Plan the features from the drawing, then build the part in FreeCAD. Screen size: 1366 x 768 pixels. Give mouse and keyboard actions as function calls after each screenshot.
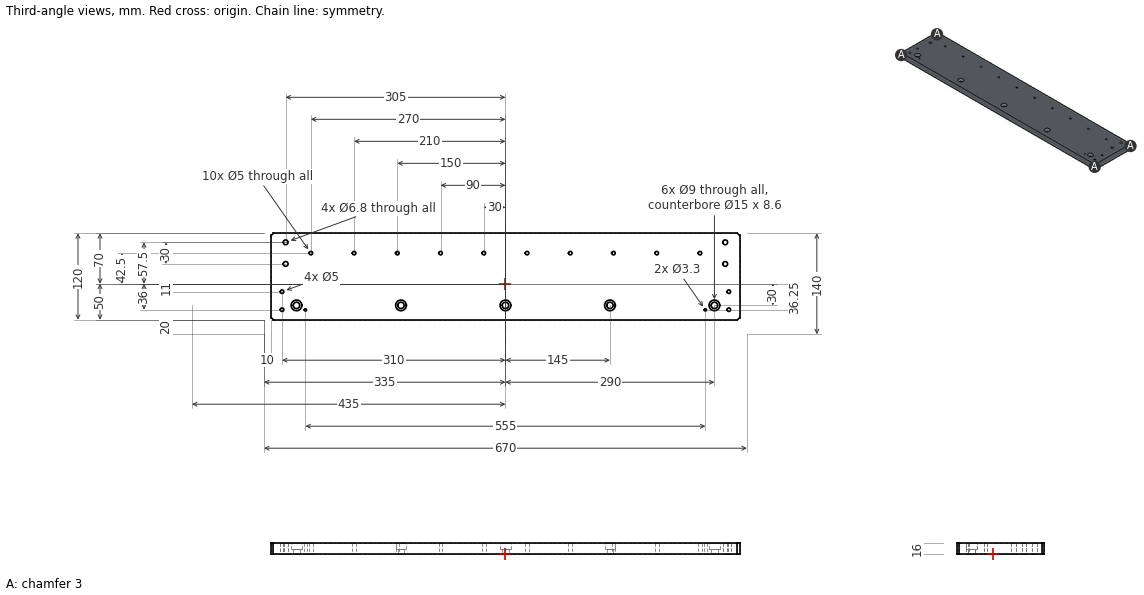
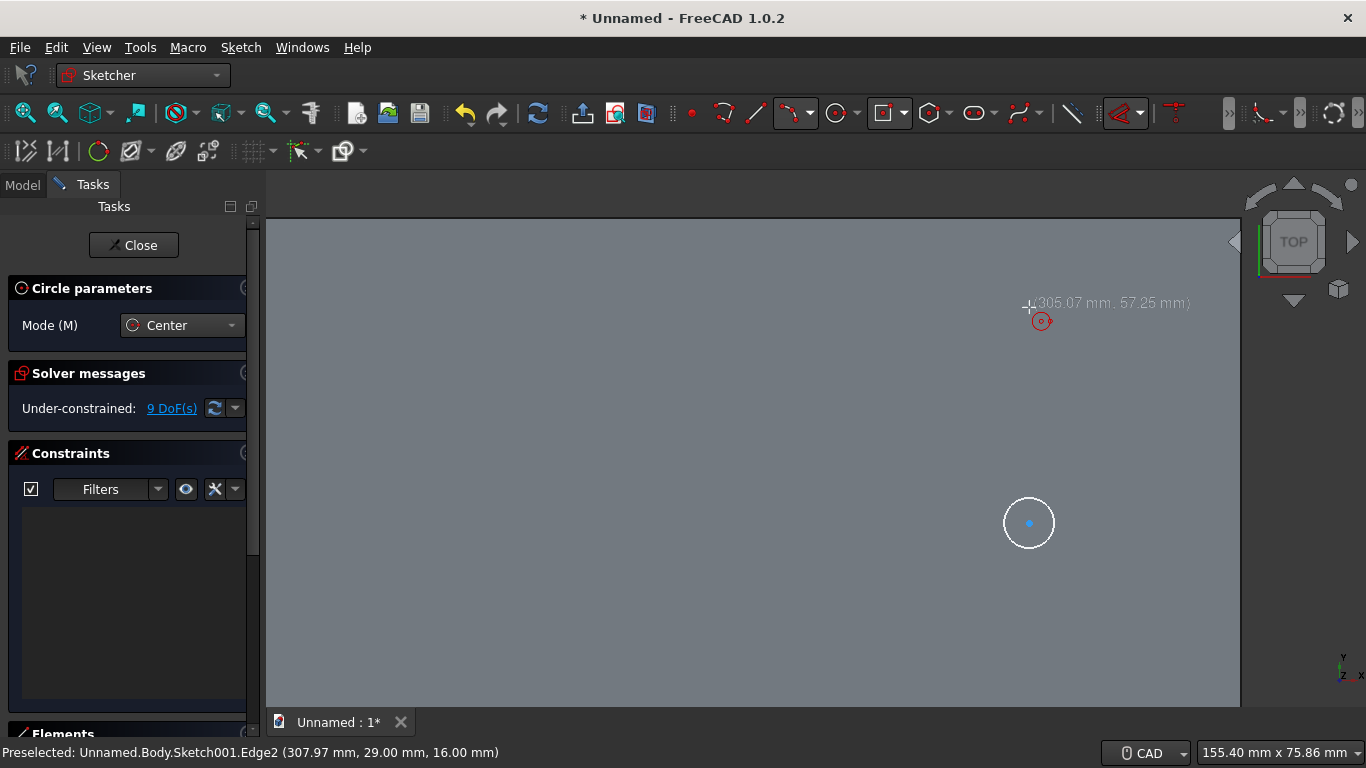
scroll(1041, 429, down, 10)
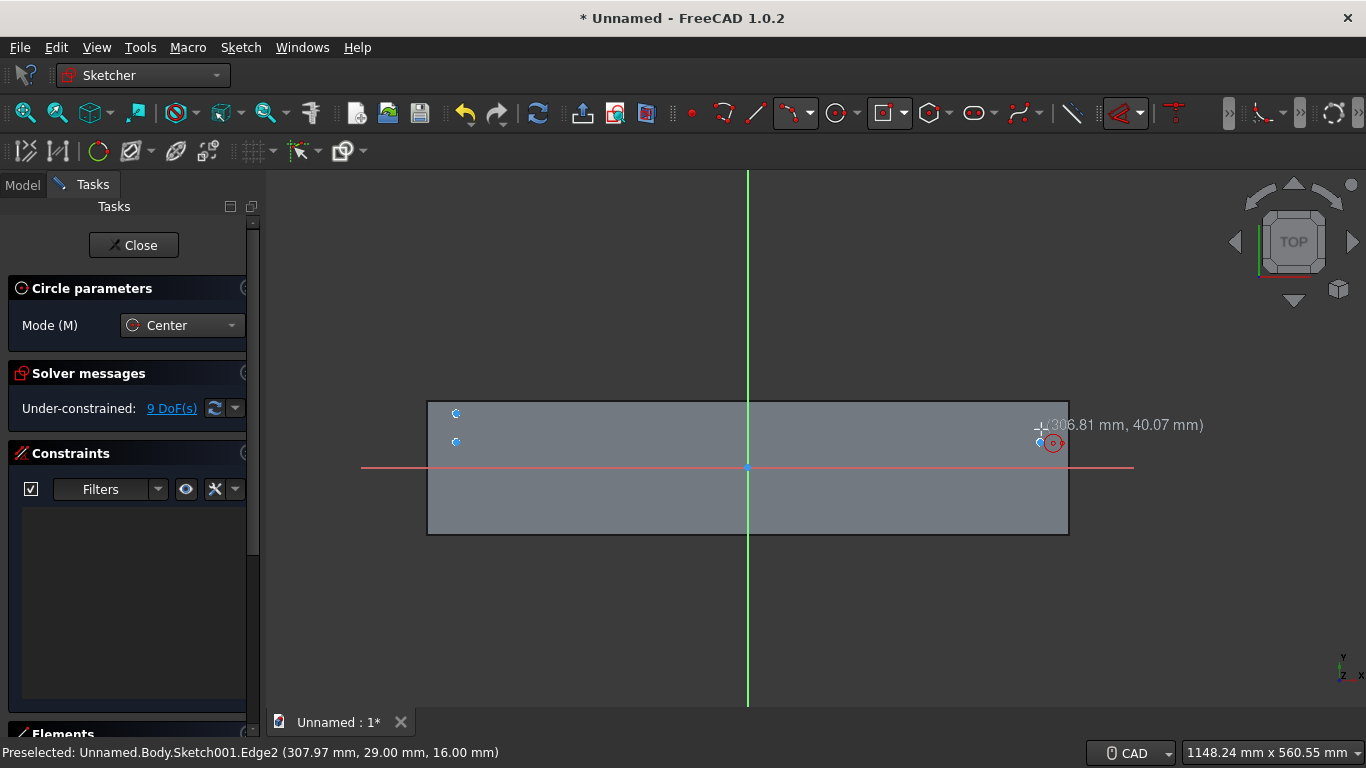
click(1040, 413)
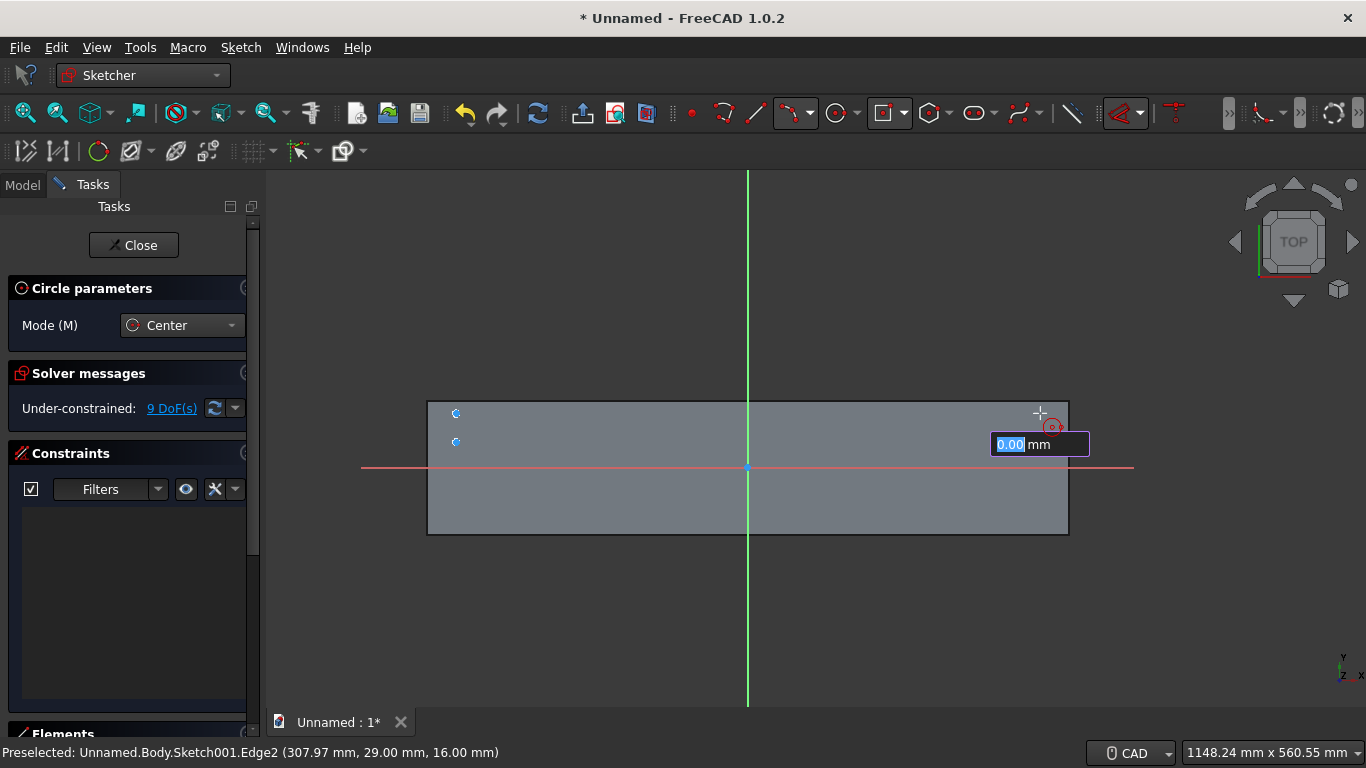
scroll(1042, 411, up, 8)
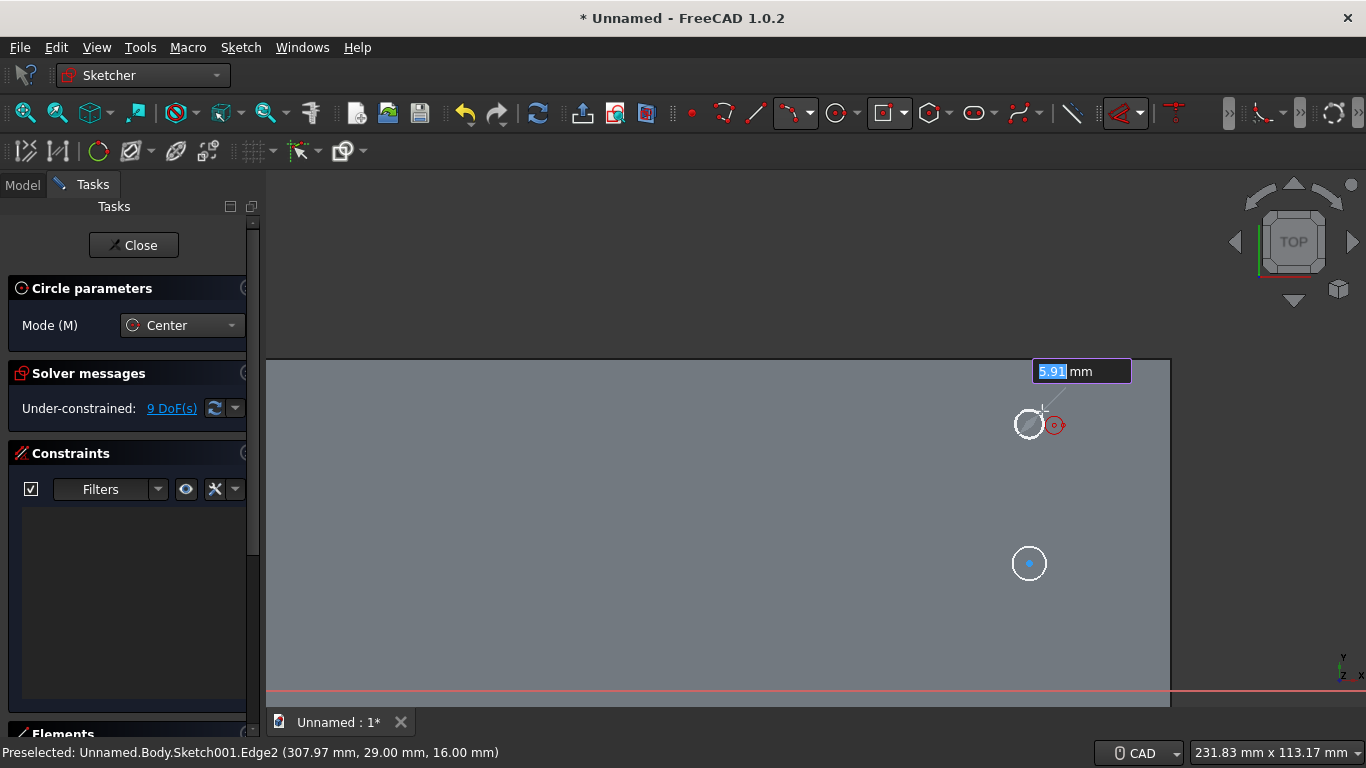
click(1040, 407)
key(Escape)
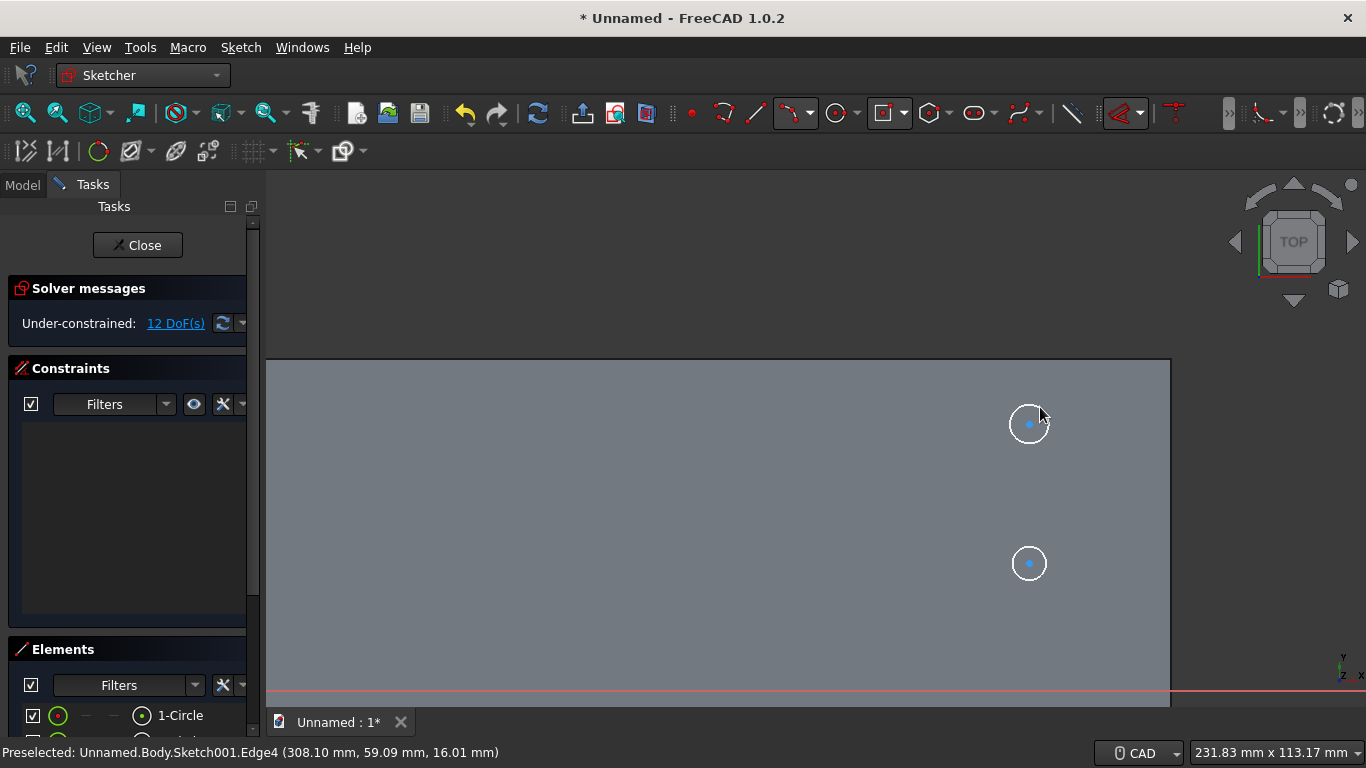
scroll(1042, 411, down, 8)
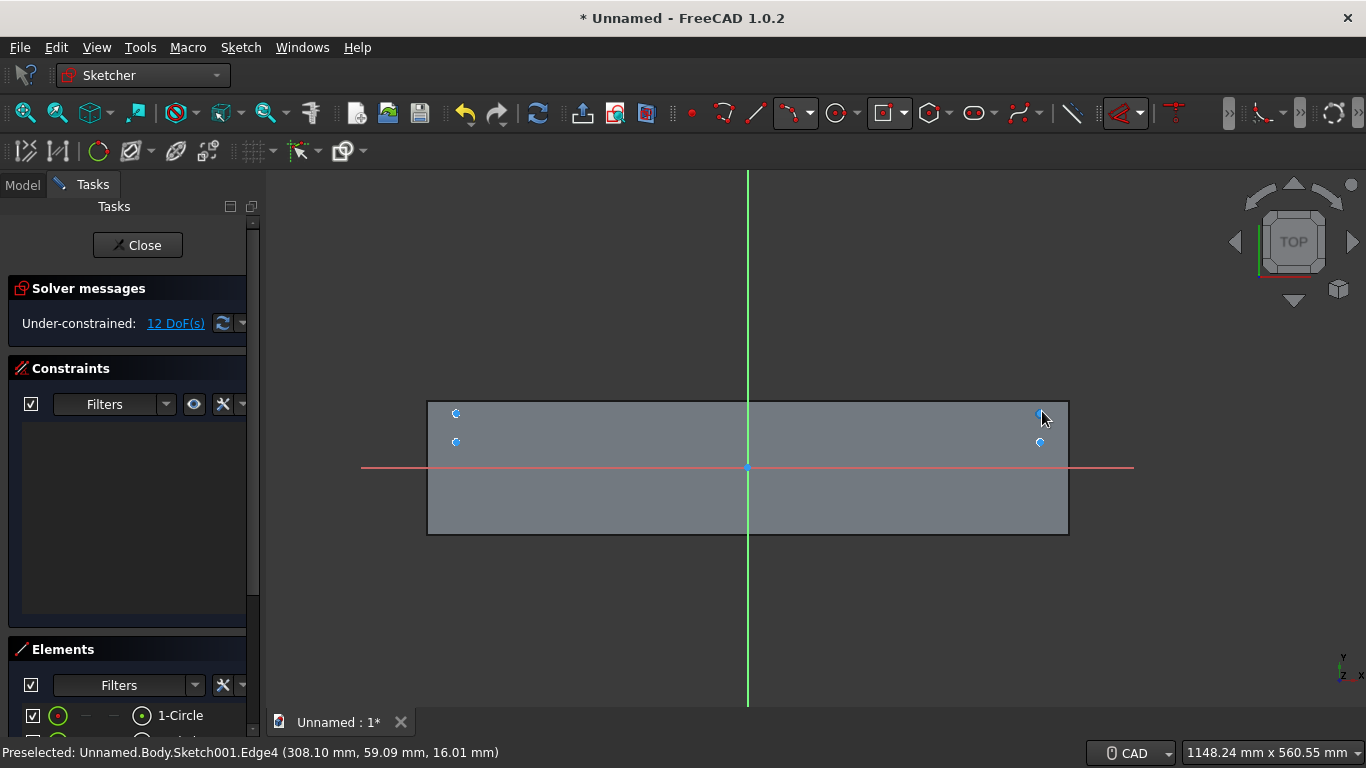
scroll(458, 411, up, 8)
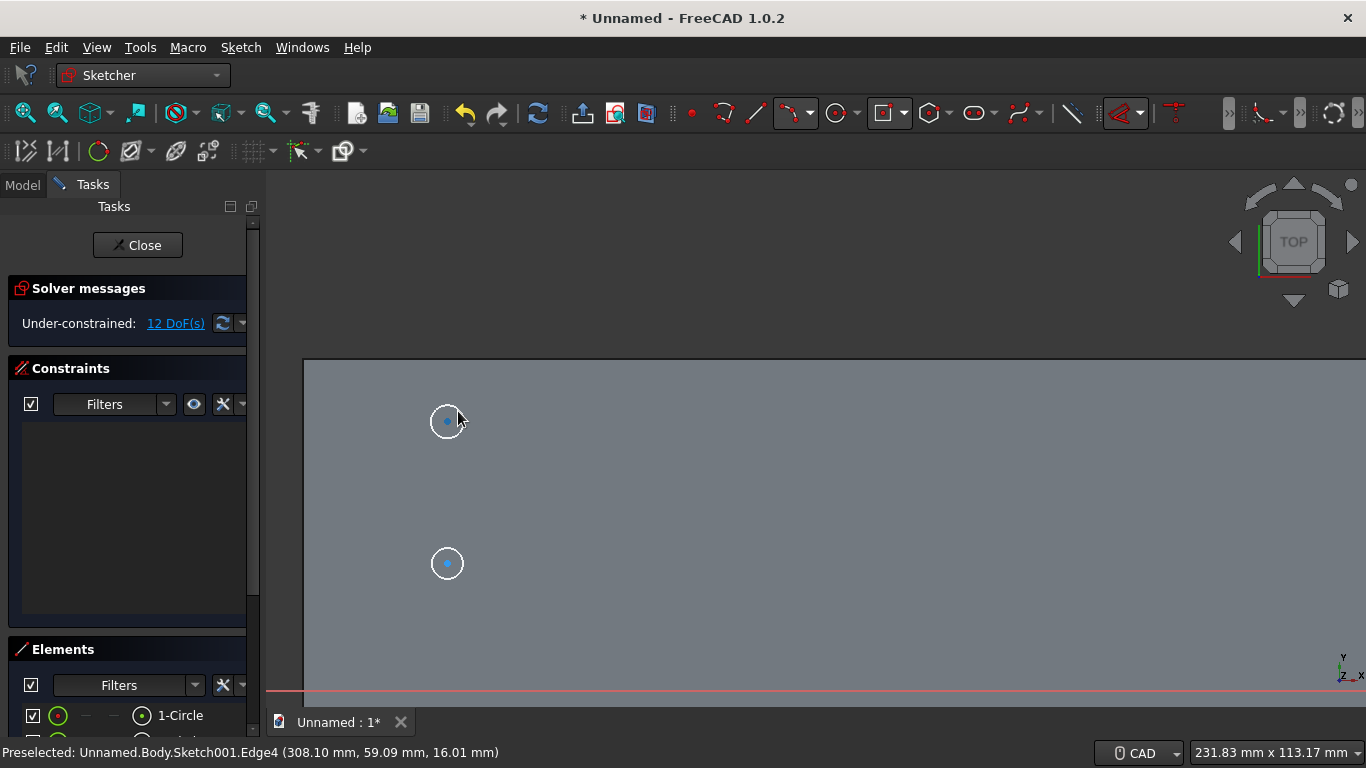
click(459, 410)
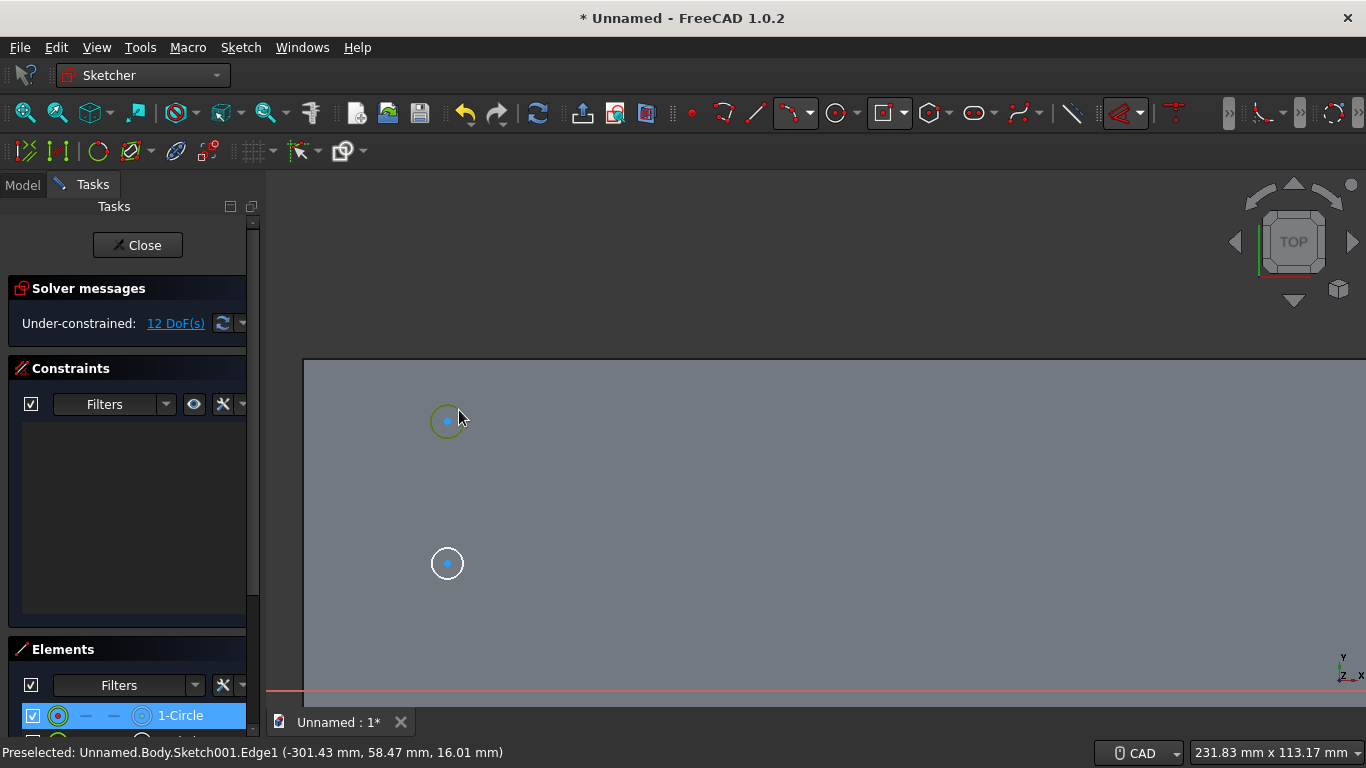
click(458, 552)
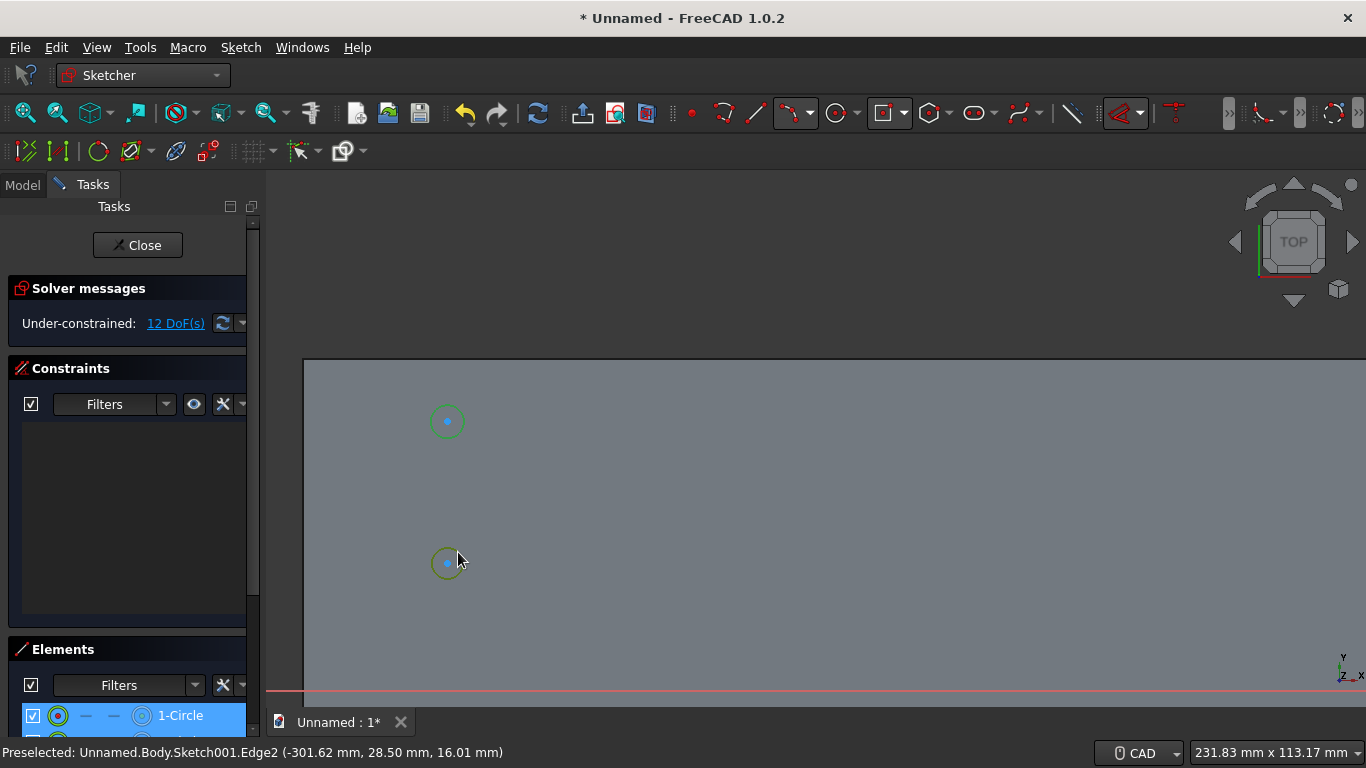
scroll(458, 411, down, 8)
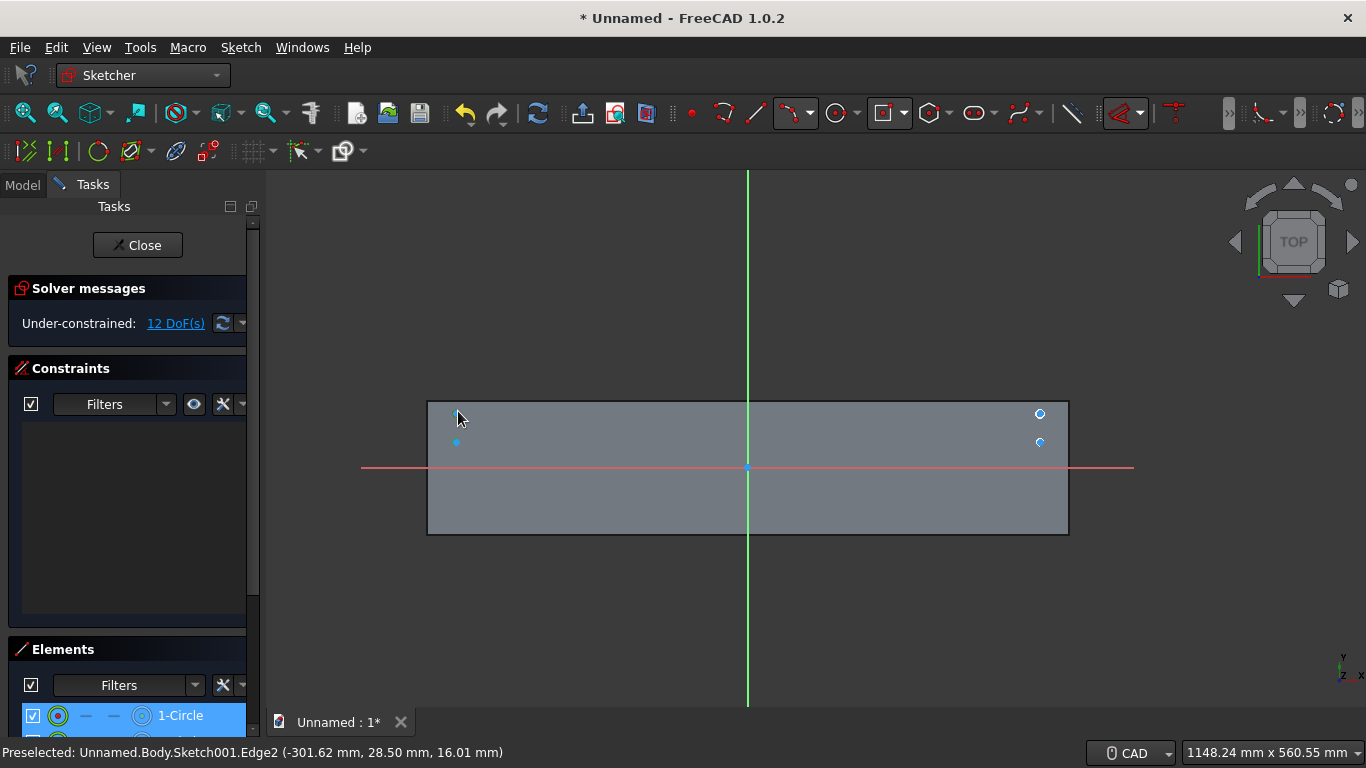
scroll(1042, 440, up, 8)